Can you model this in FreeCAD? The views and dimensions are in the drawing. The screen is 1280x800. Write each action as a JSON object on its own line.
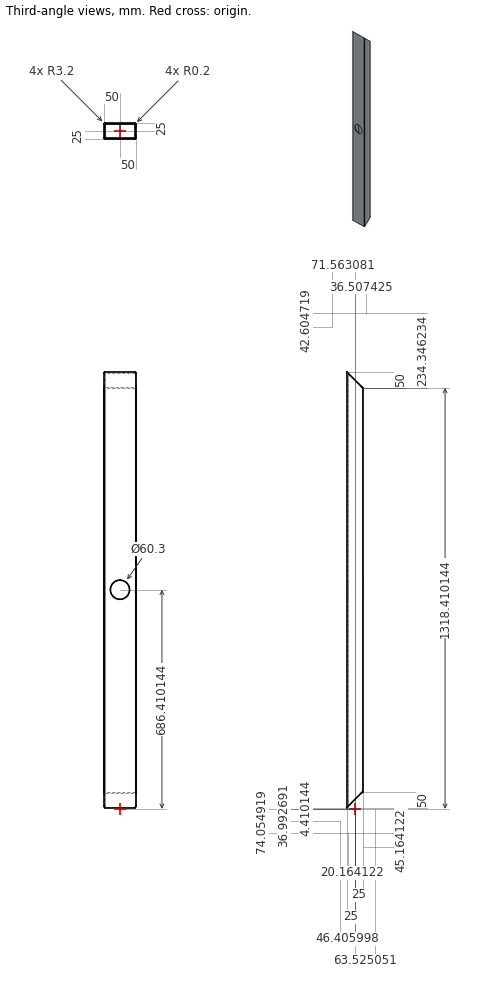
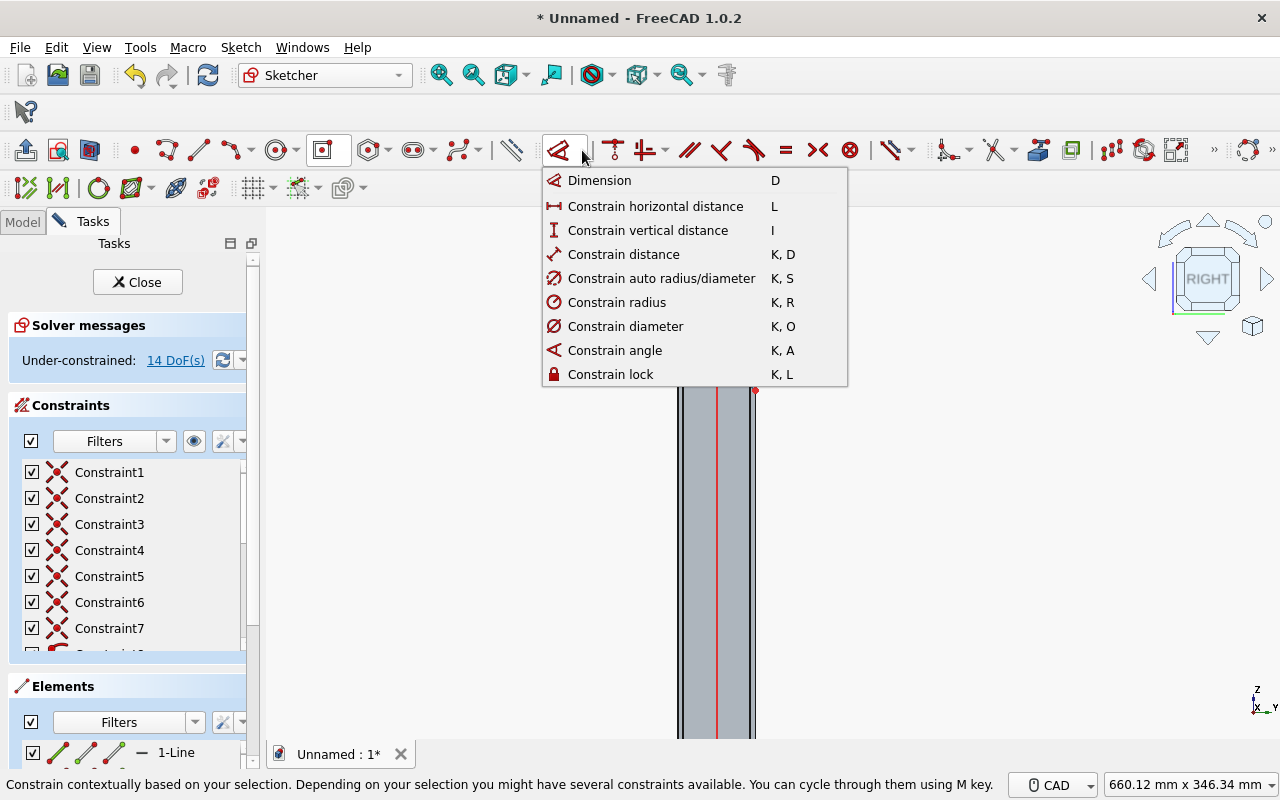
{"action": "left_click", "coordinate": [695, 230]}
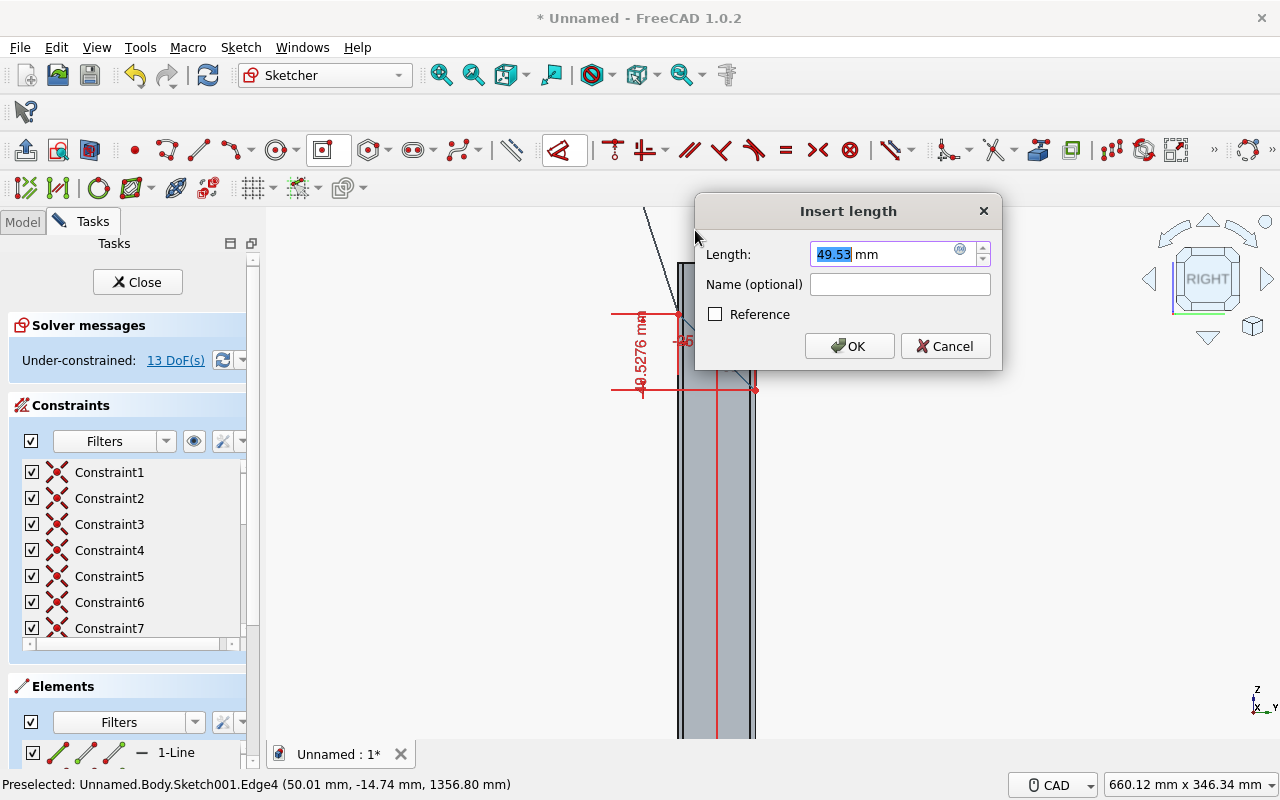
{"action": "type", "text": "50"}
{"action": "key", "text": "Return"}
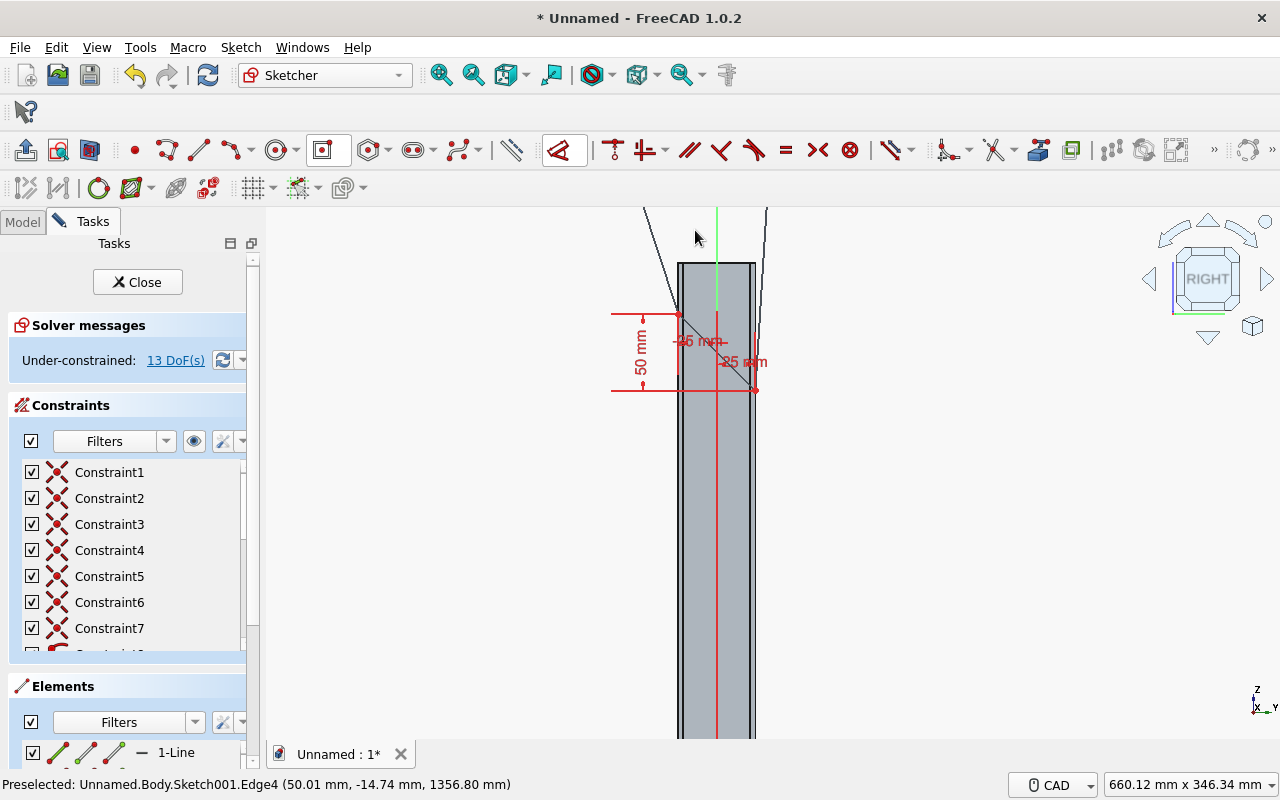
{"action": "scroll", "coordinate": [704, 342], "scroll_direction": "down", "scroll_amount": 10}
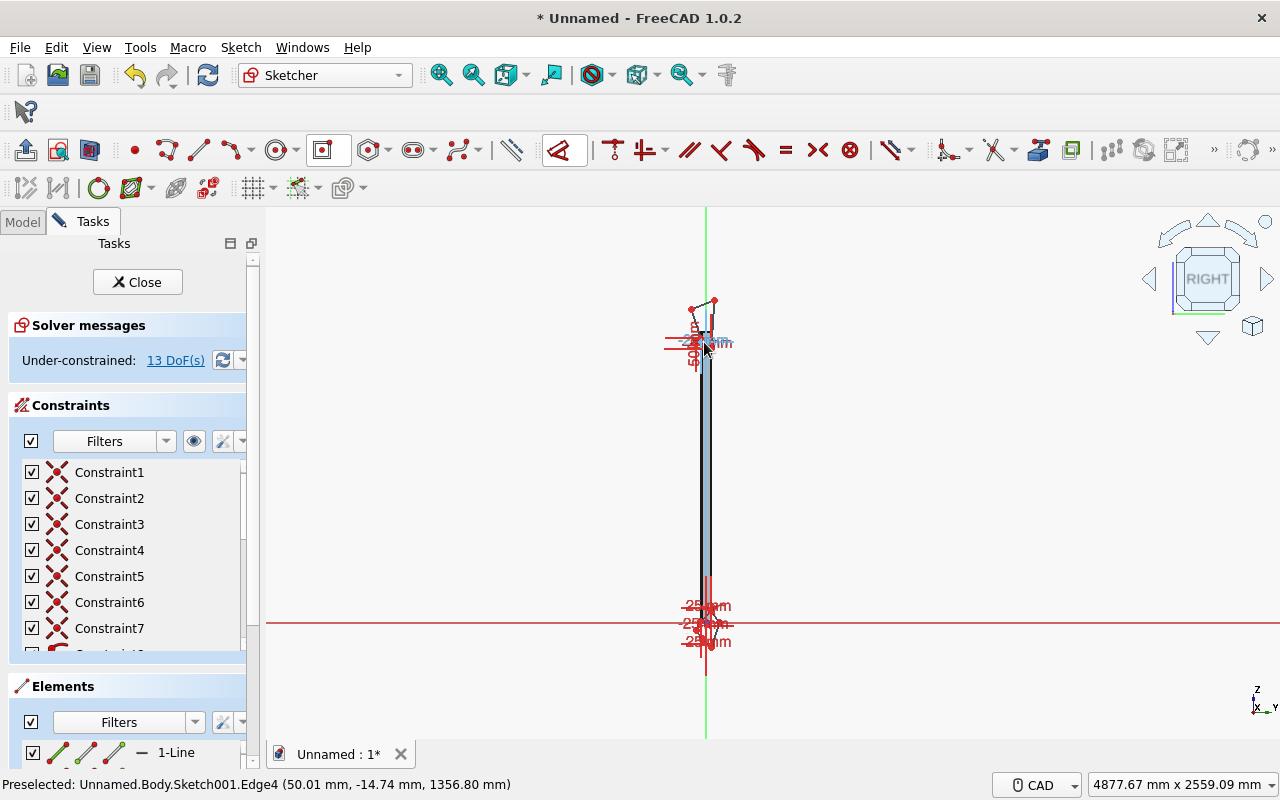
{"action": "scroll", "coordinate": [708, 615], "scroll_direction": "up", "scroll_amount": 10}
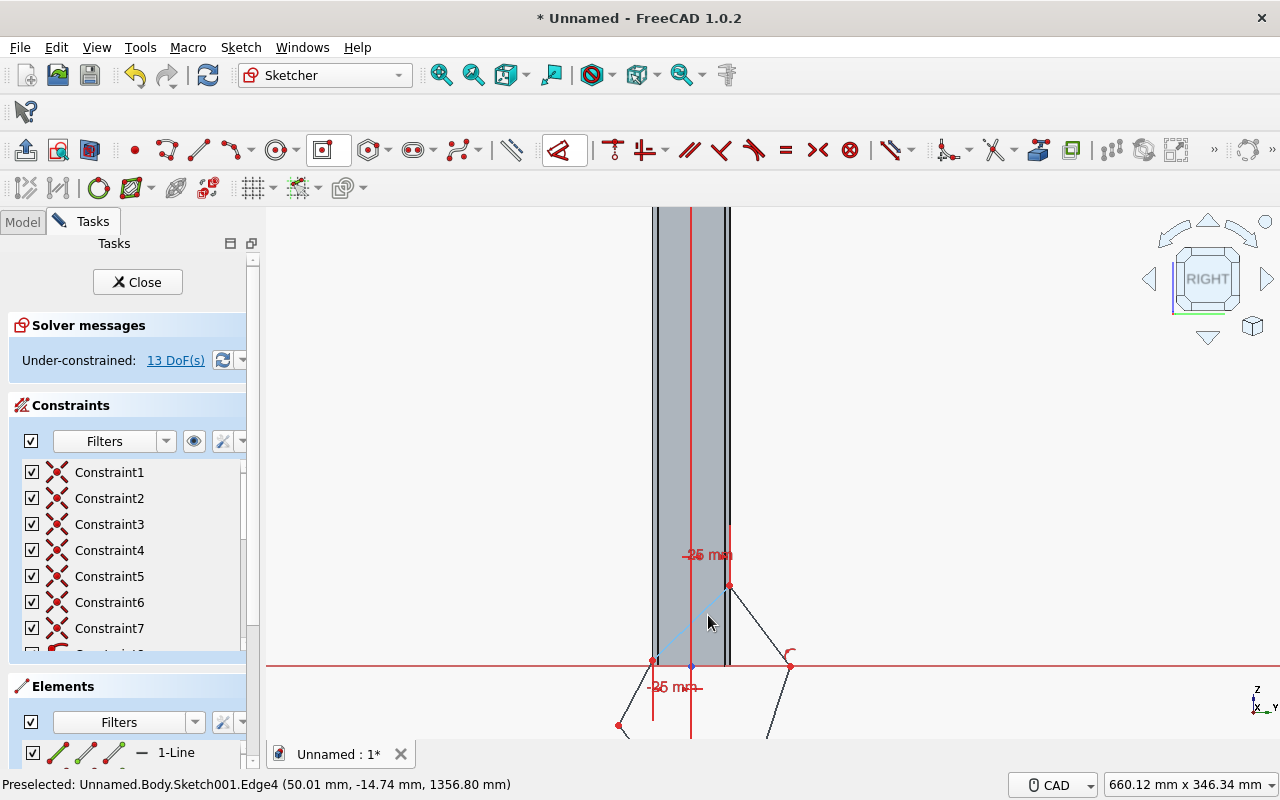
{"action": "left_click", "coordinate": [707, 608]}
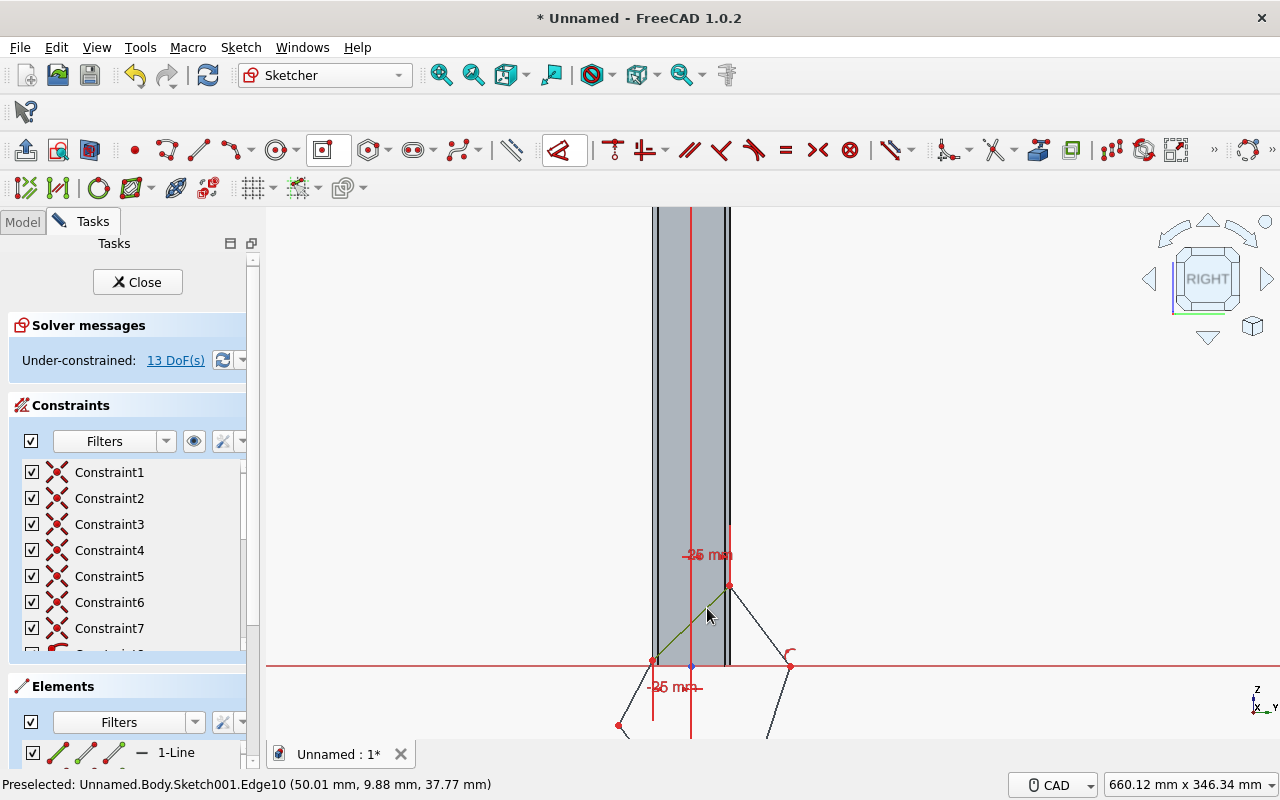
{"action": "key", "text": "i"}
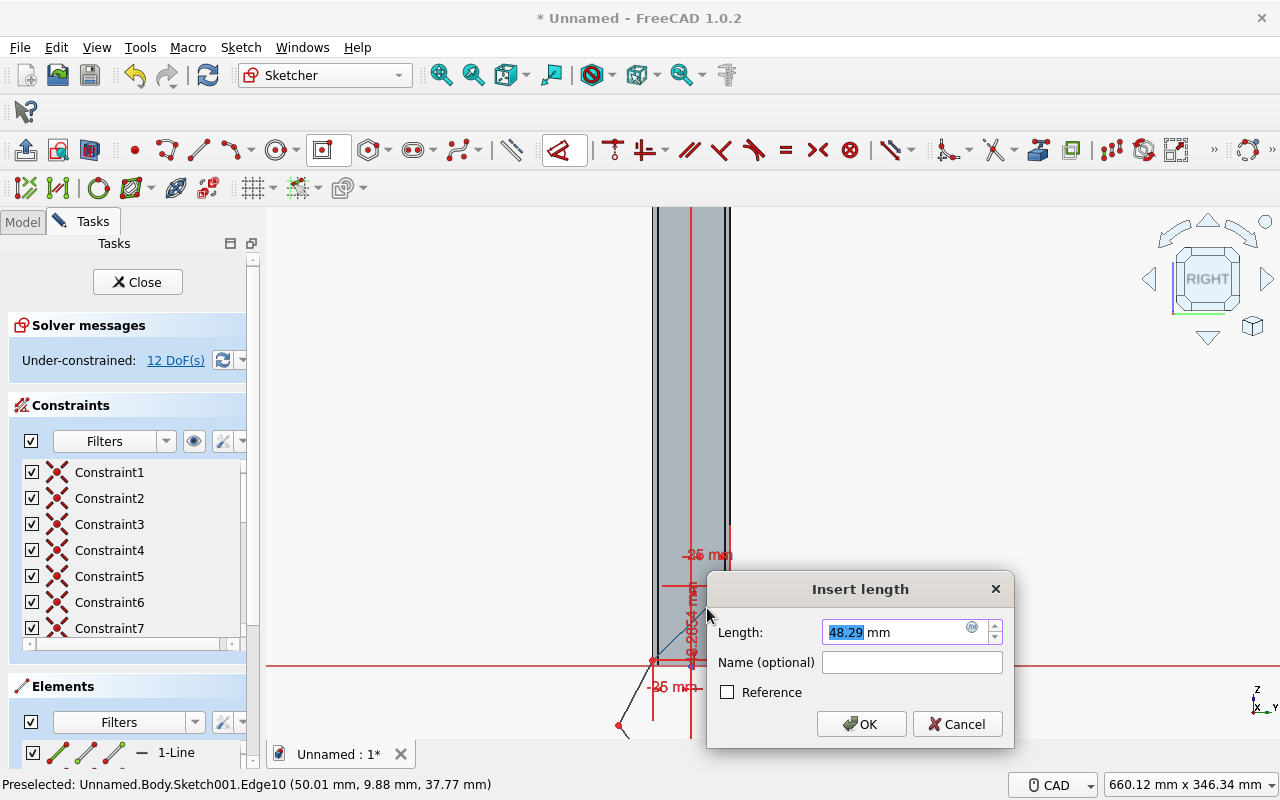
{"action": "type", "text": "50"}
{"action": "key", "text": "Return"}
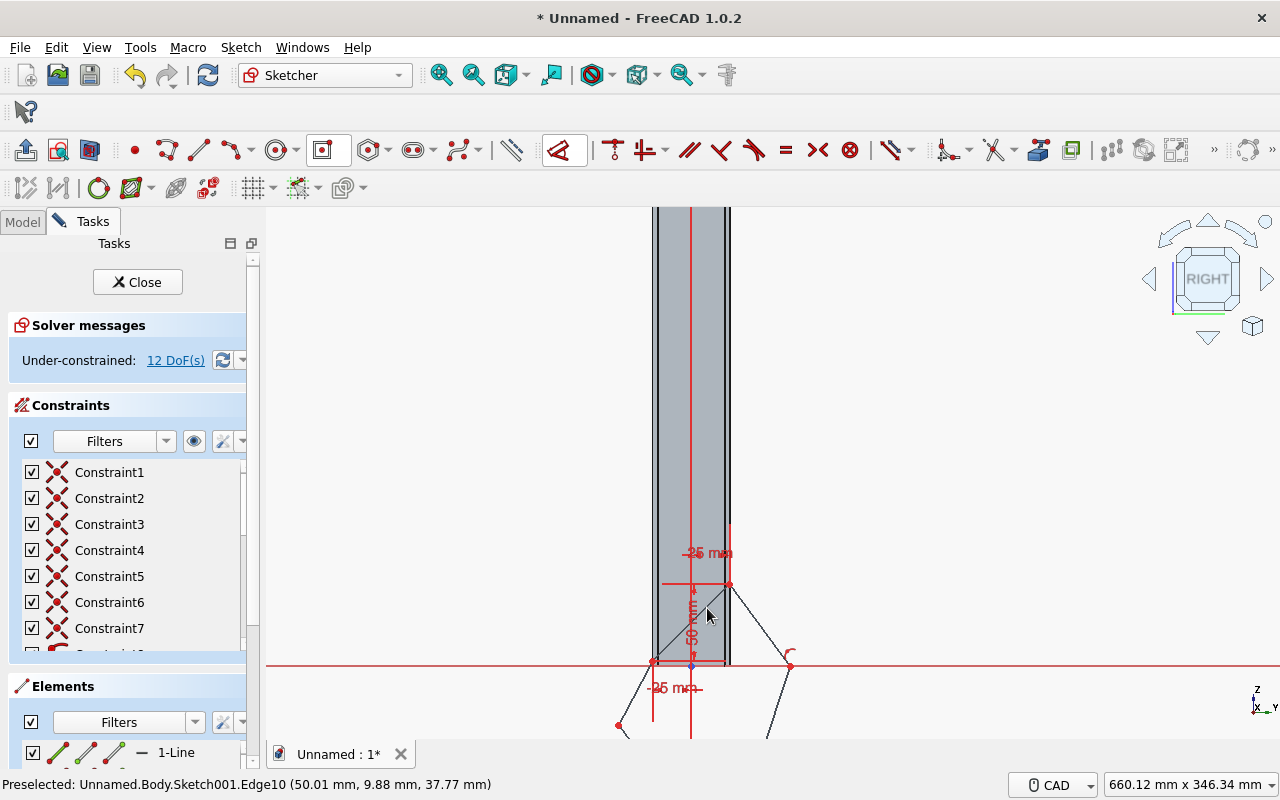
{"action": "scroll", "coordinate": [653, 661], "scroll_direction": "up", "scroll_amount": 9}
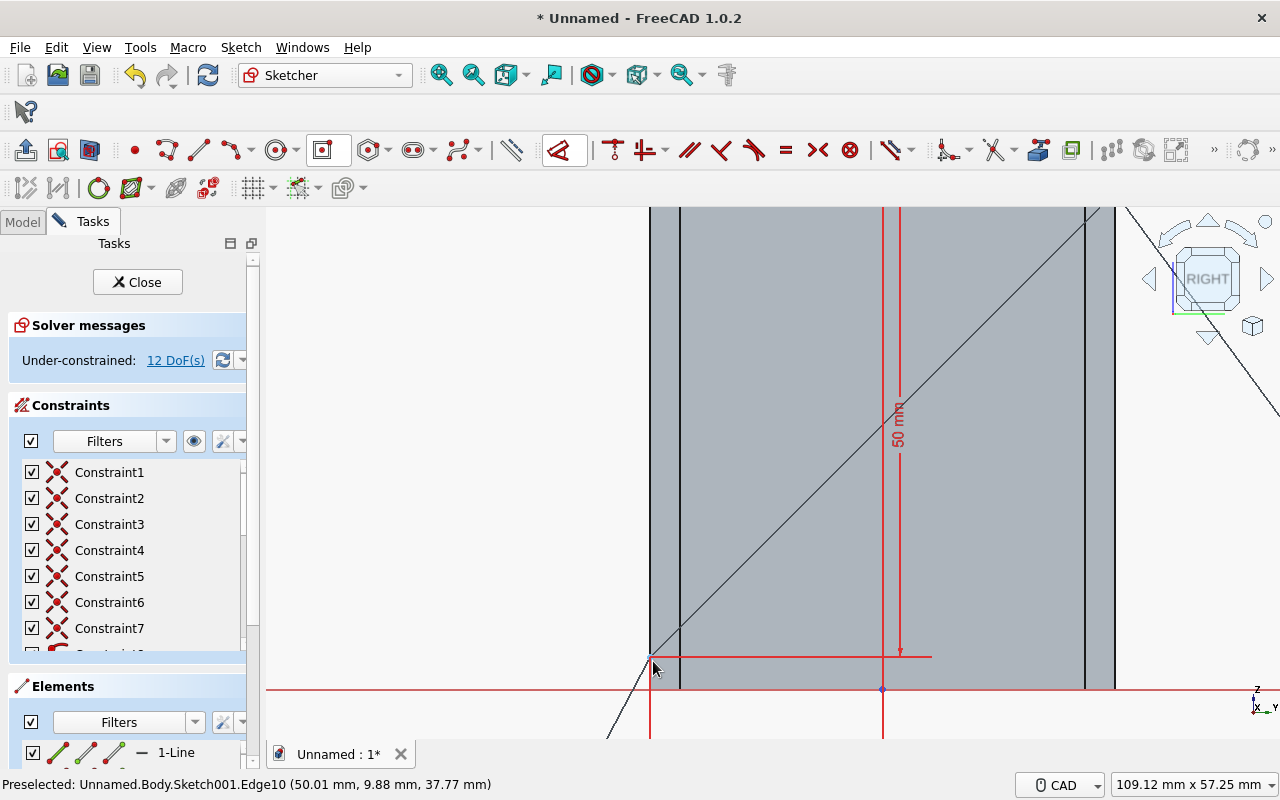
{"action": "left_click", "coordinate": [650, 657]}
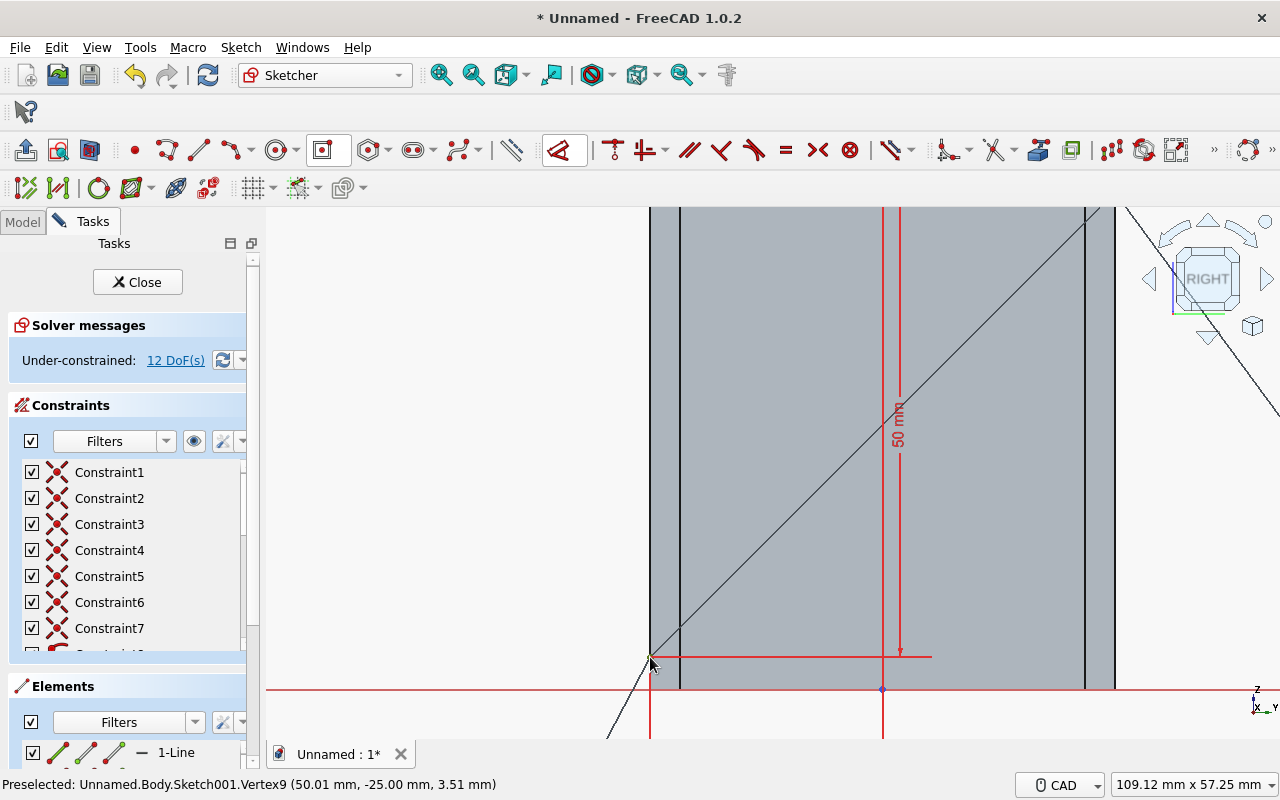
{"action": "left_click", "coordinate": [582, 150]}